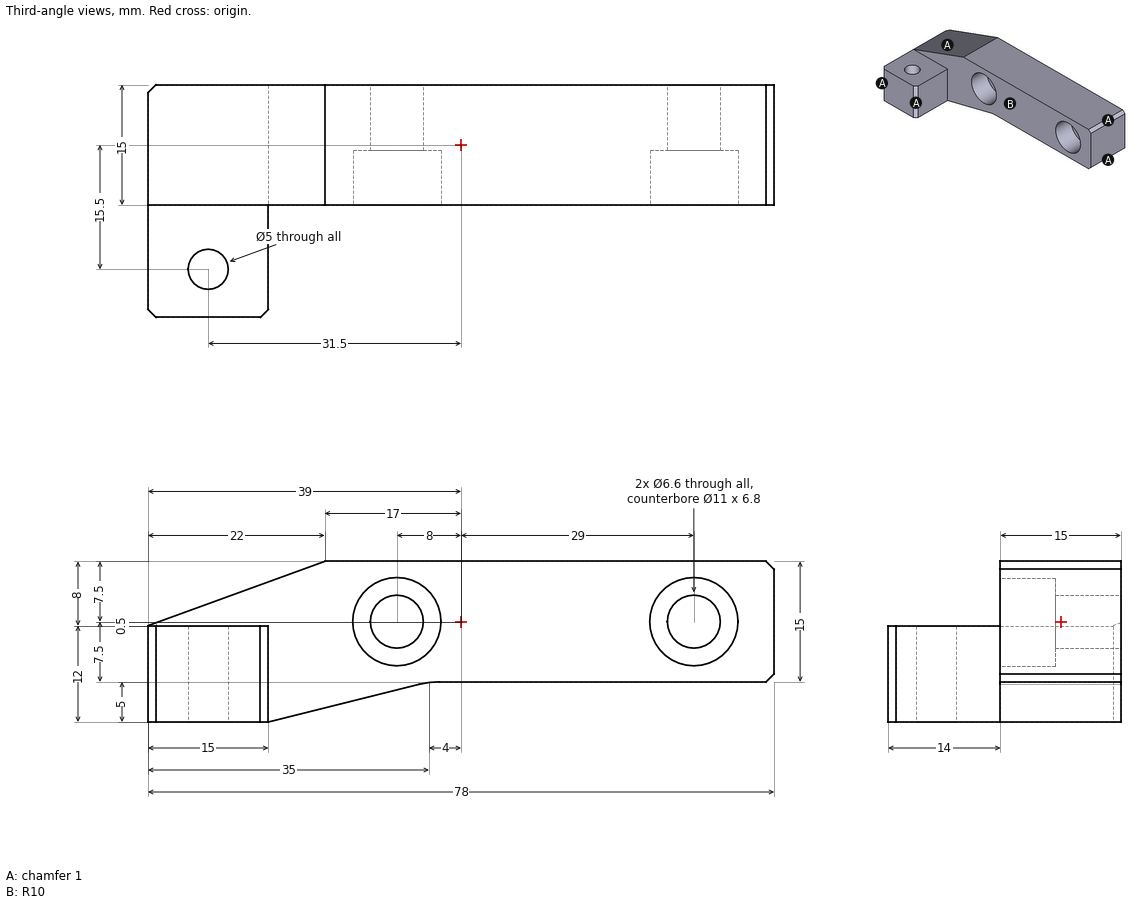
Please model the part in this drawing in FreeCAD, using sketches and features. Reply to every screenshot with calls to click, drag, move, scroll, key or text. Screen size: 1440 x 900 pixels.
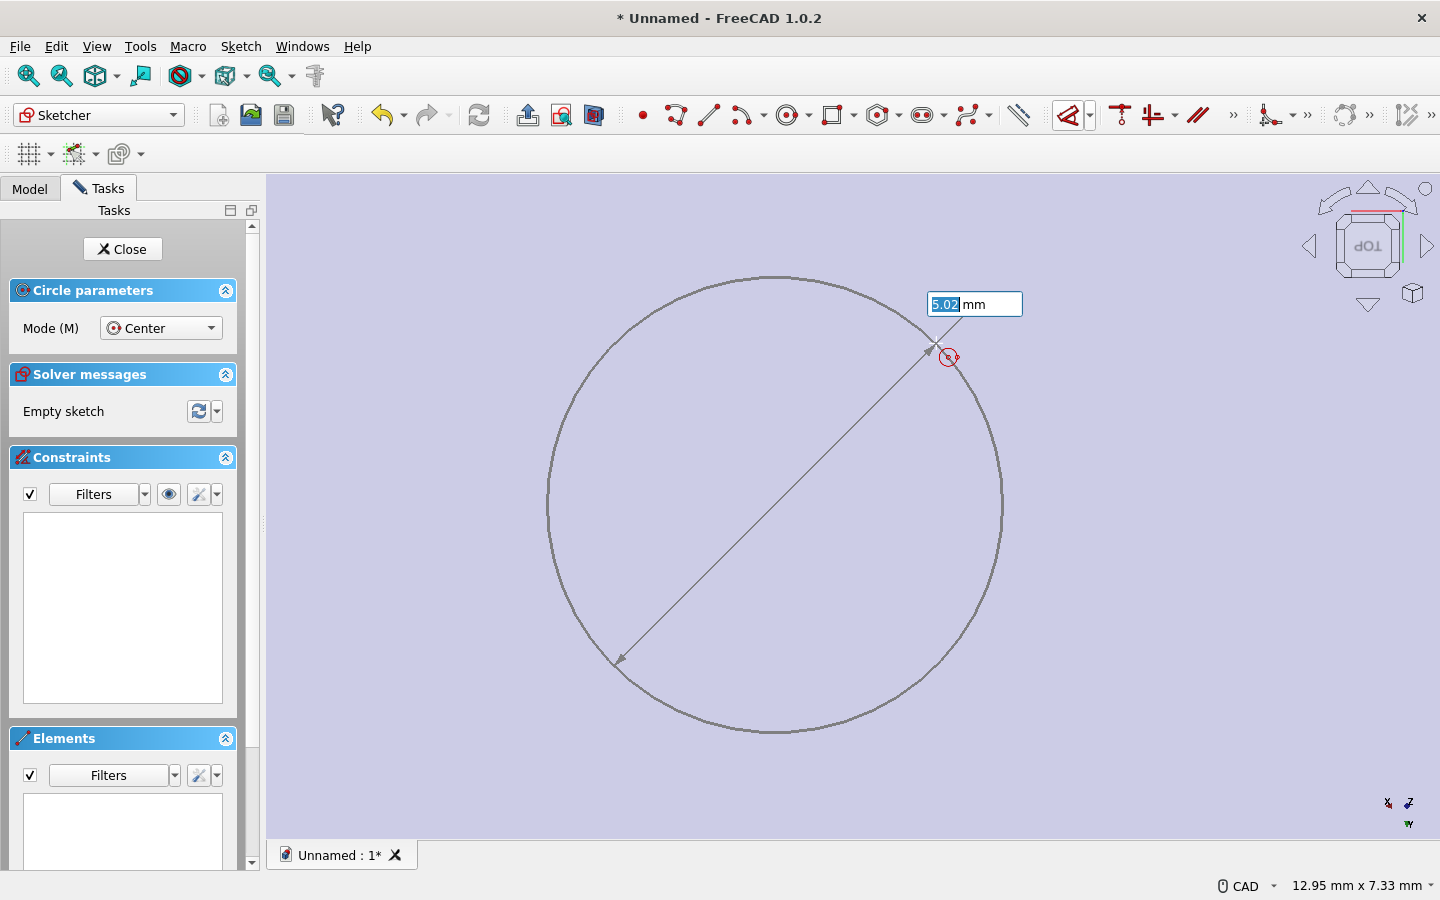
text(5)
key(Return)
key(Escape)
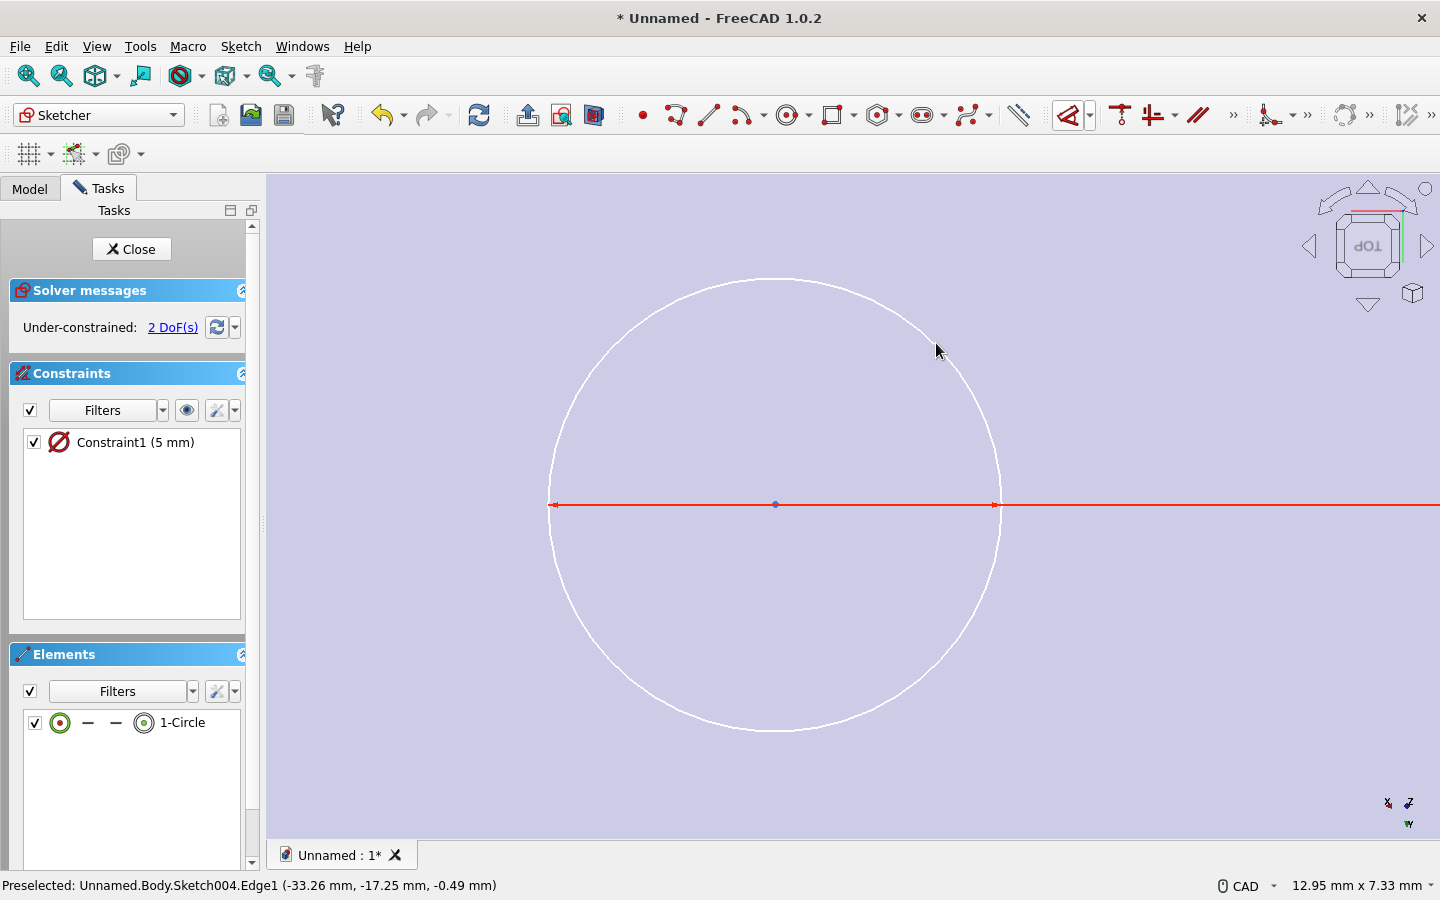
click(775, 505)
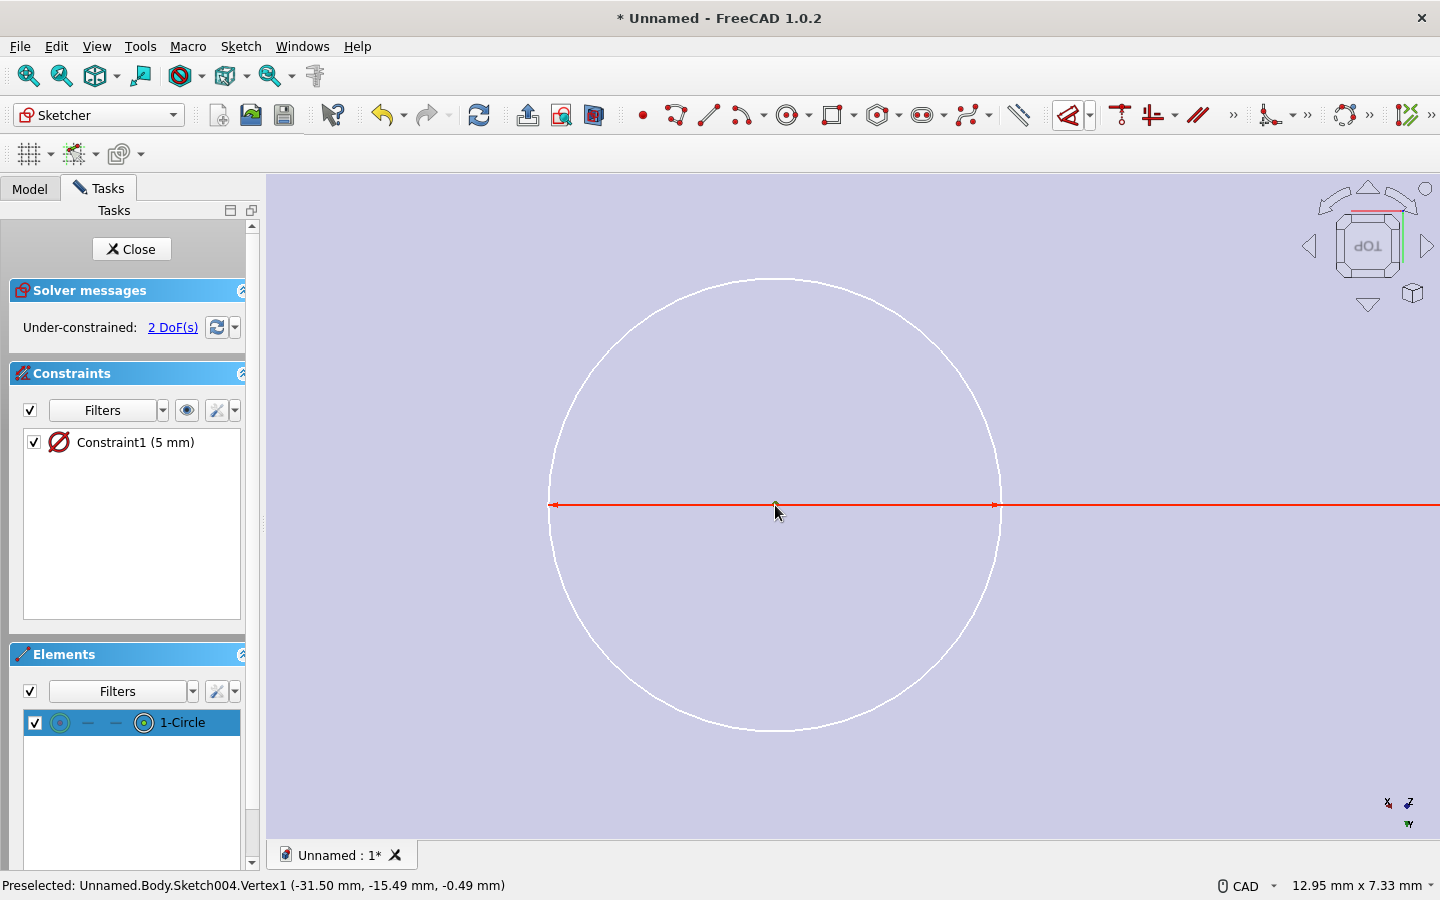
click(1090, 116)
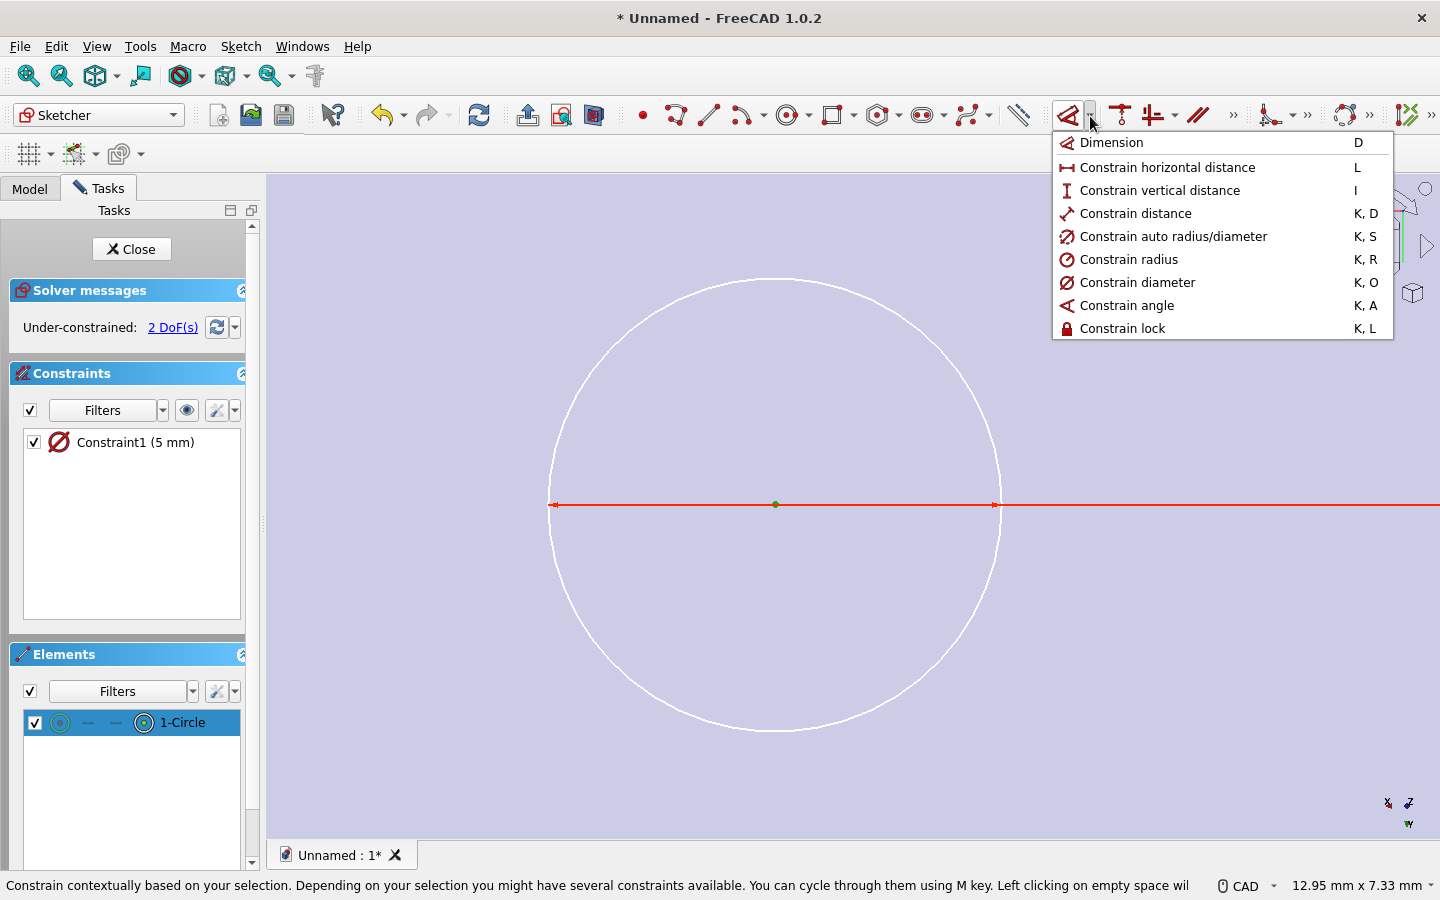
click(1223, 168)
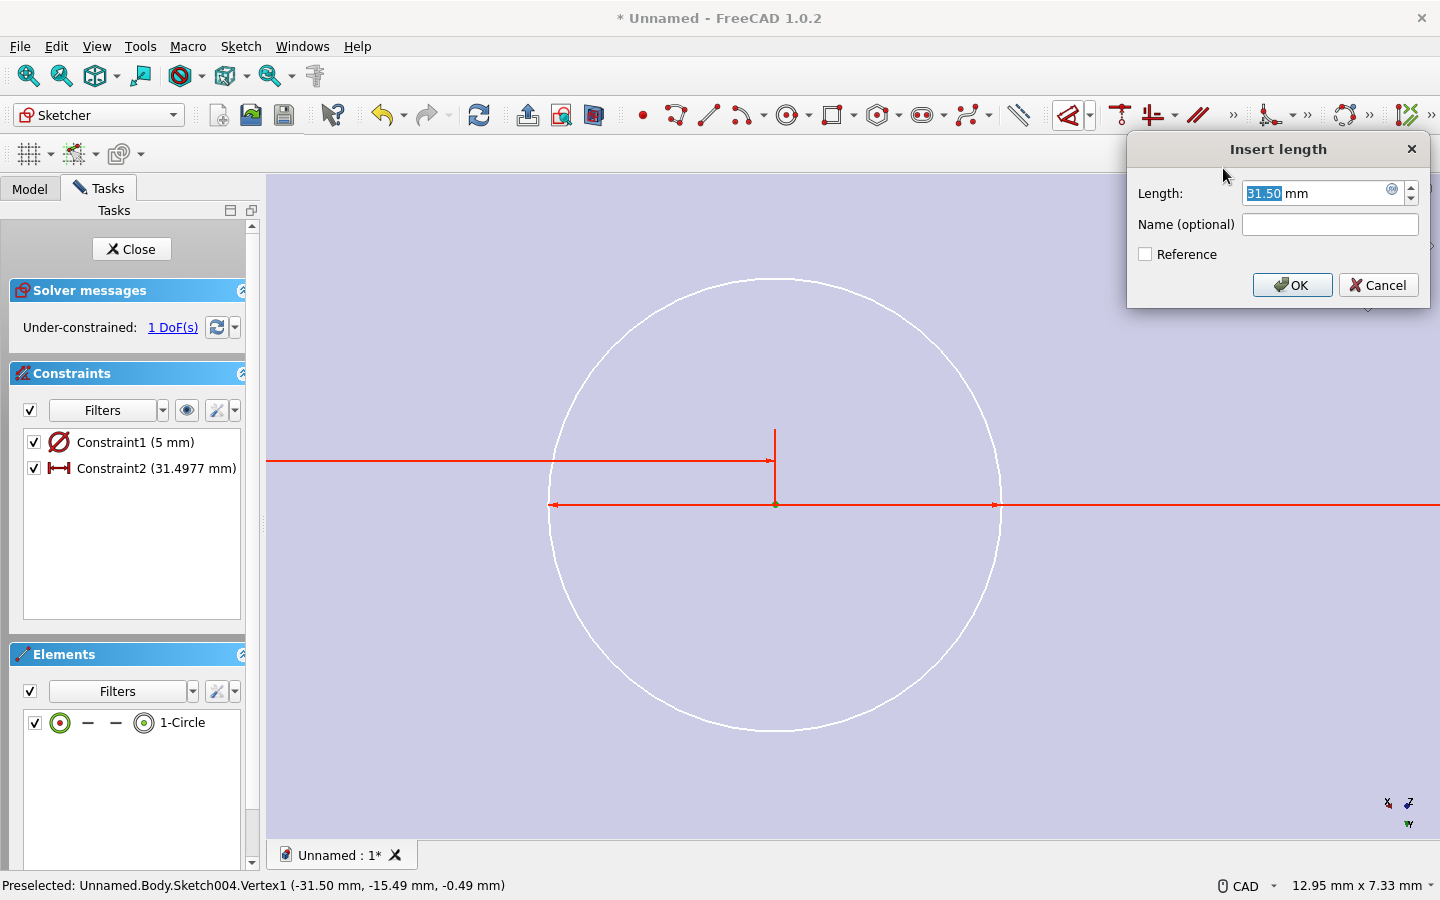
text(31.5)
key(Return)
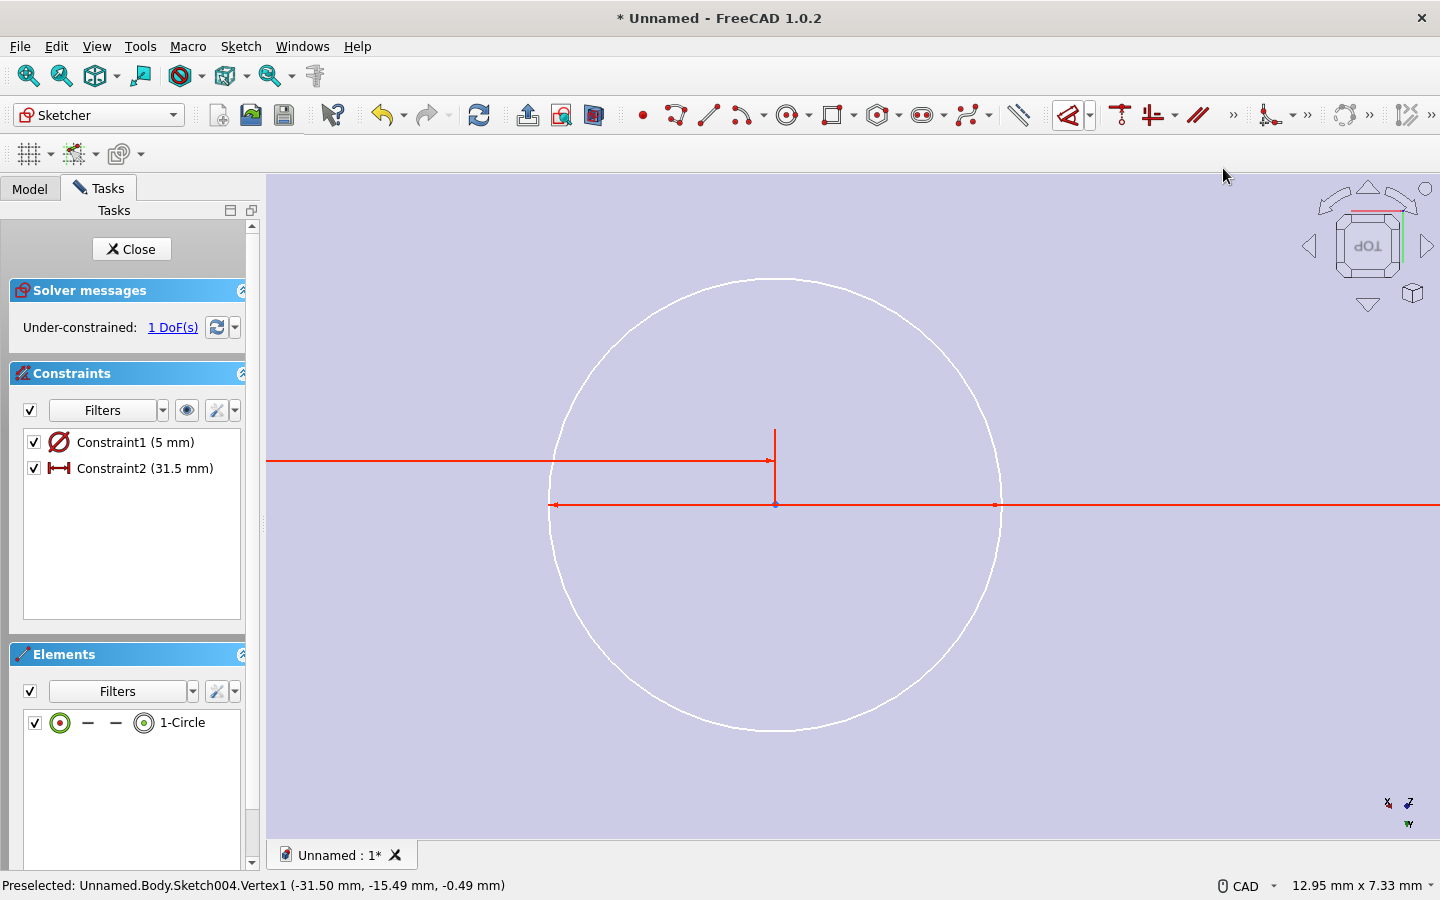
click(775, 505)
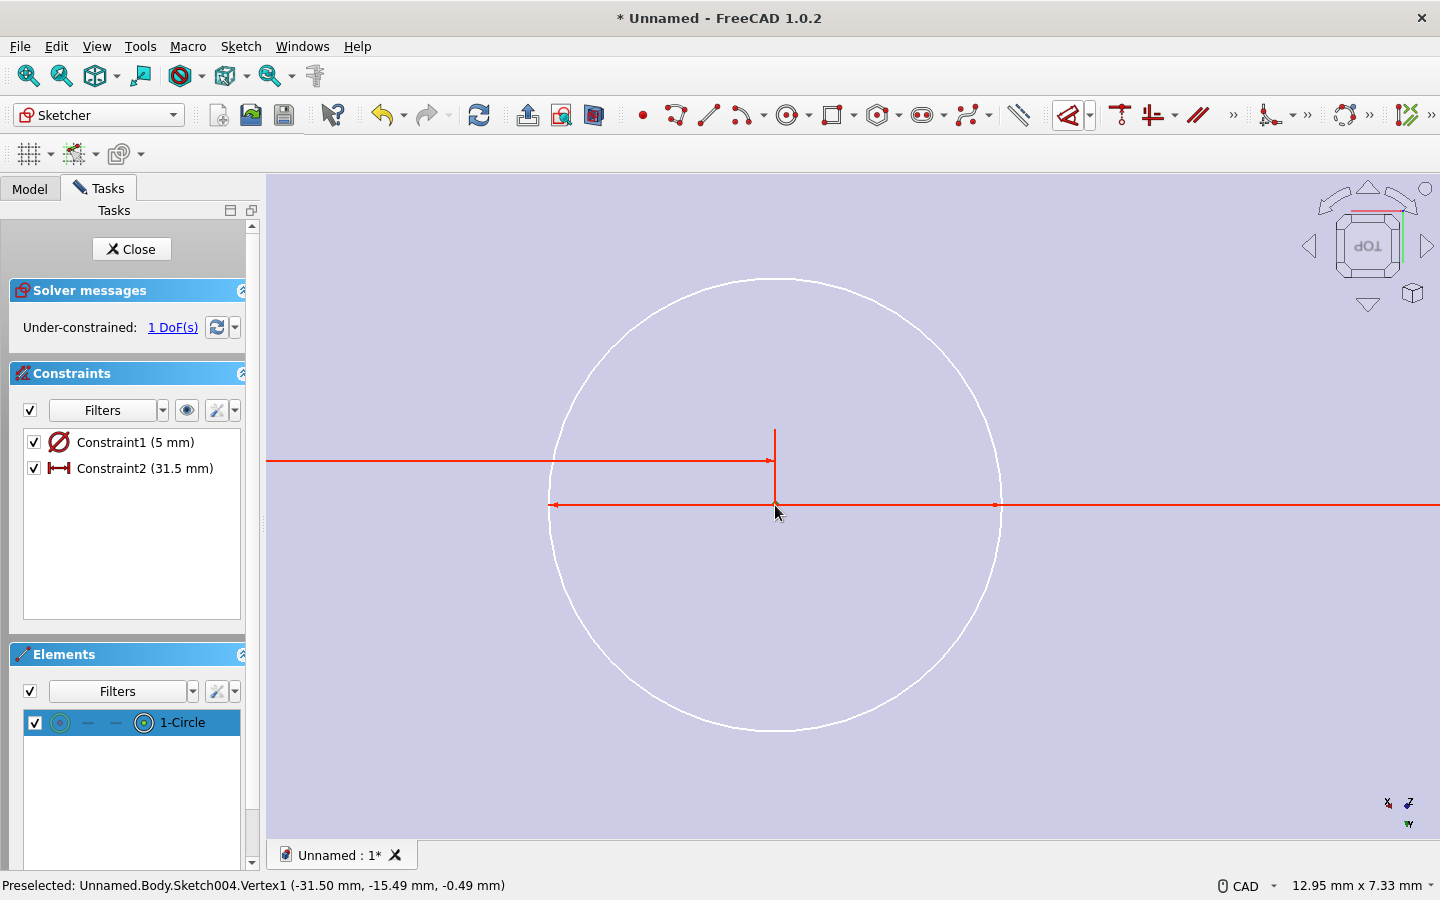
click(1090, 116)